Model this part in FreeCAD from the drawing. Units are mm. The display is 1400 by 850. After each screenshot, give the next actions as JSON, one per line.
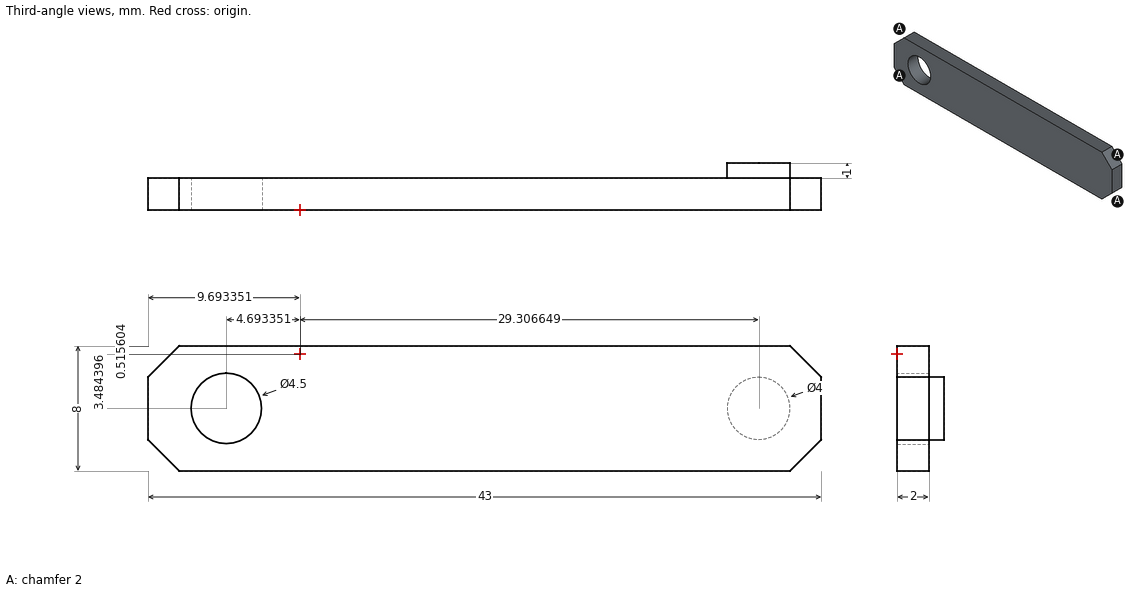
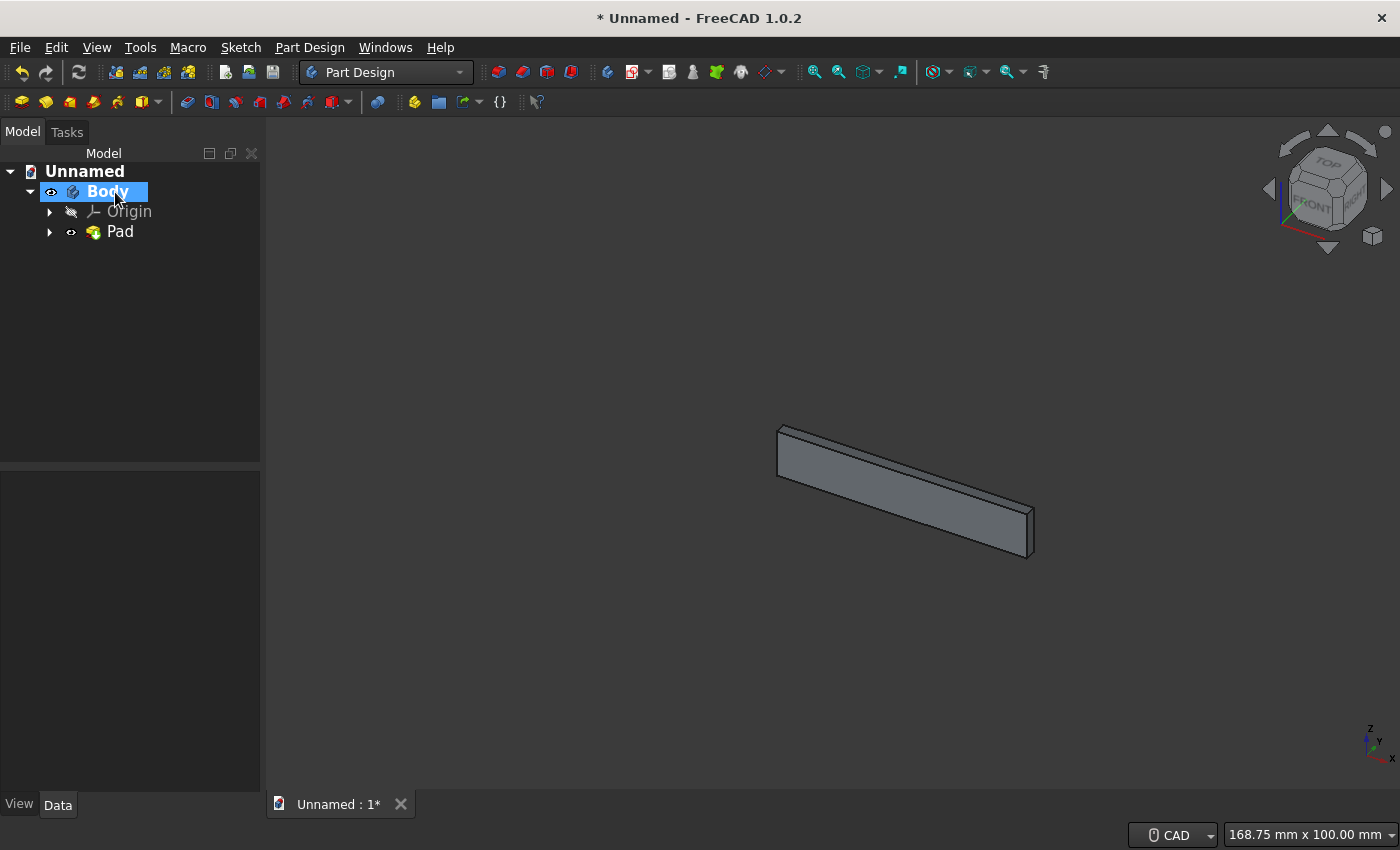
{"action": "left_click", "coordinate": [816, 72]}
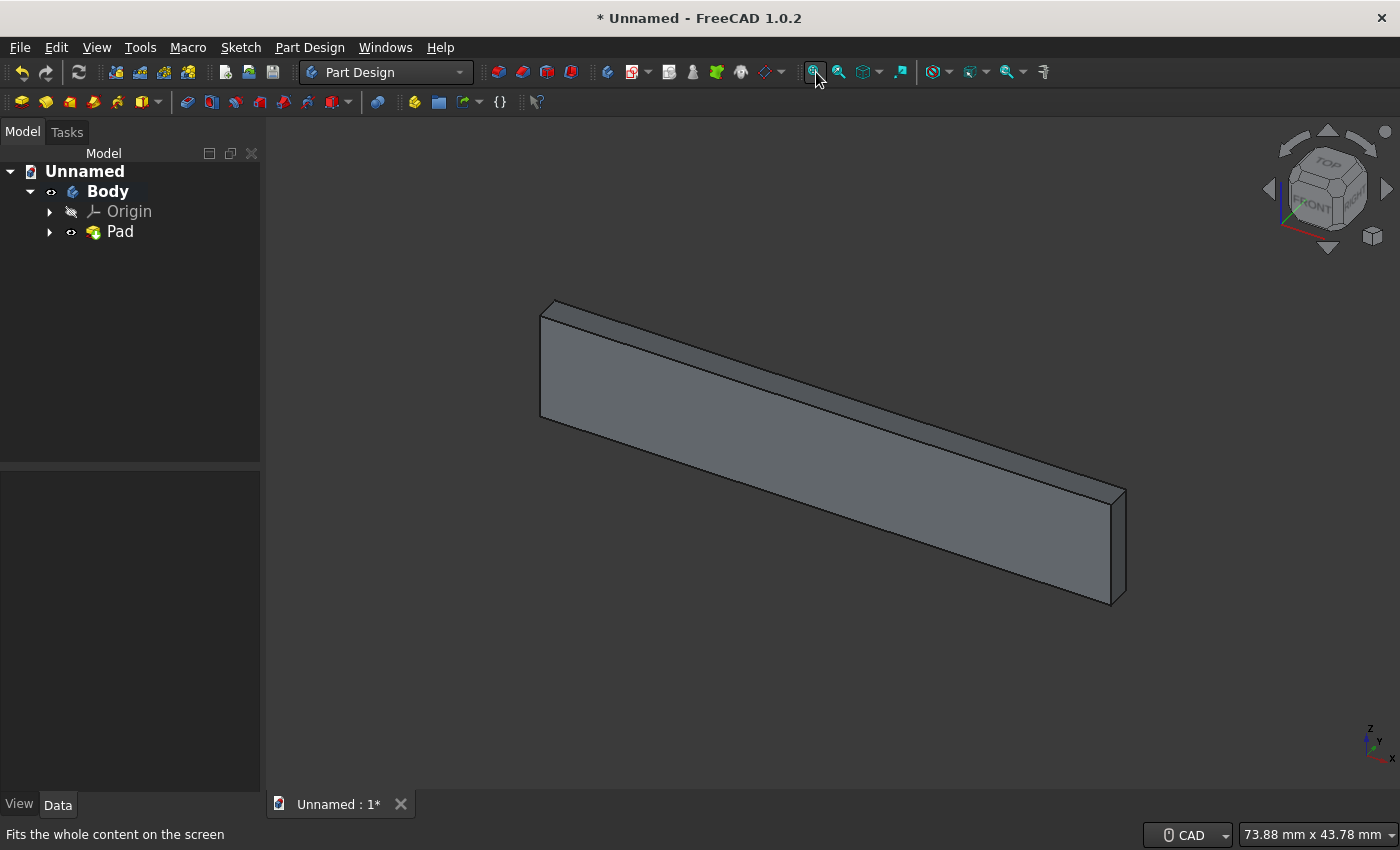
{"action": "key", "text": "4"}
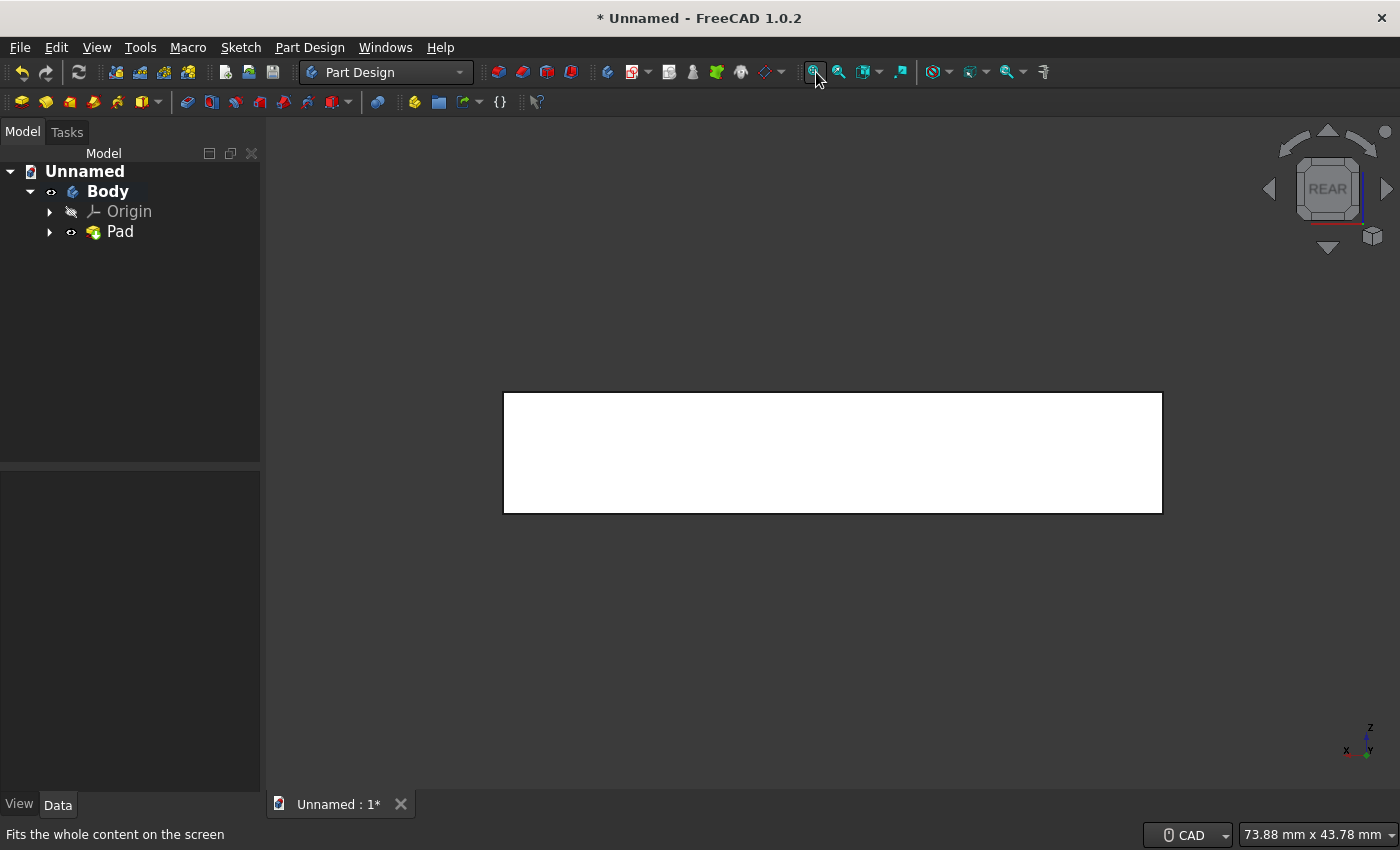
{"action": "left_click", "coordinate": [644, 452]}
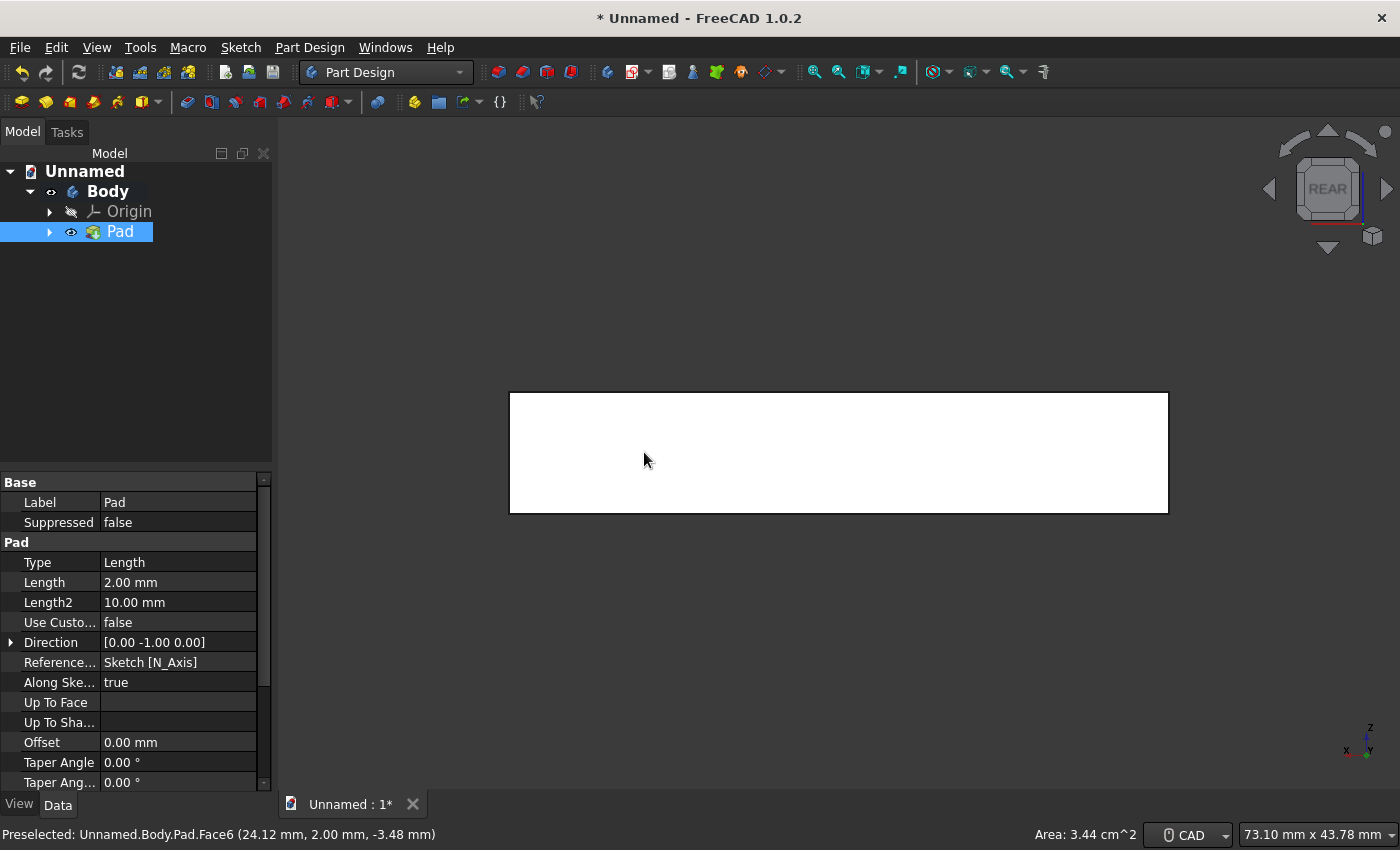
{"action": "left_click", "coordinate": [632, 72]}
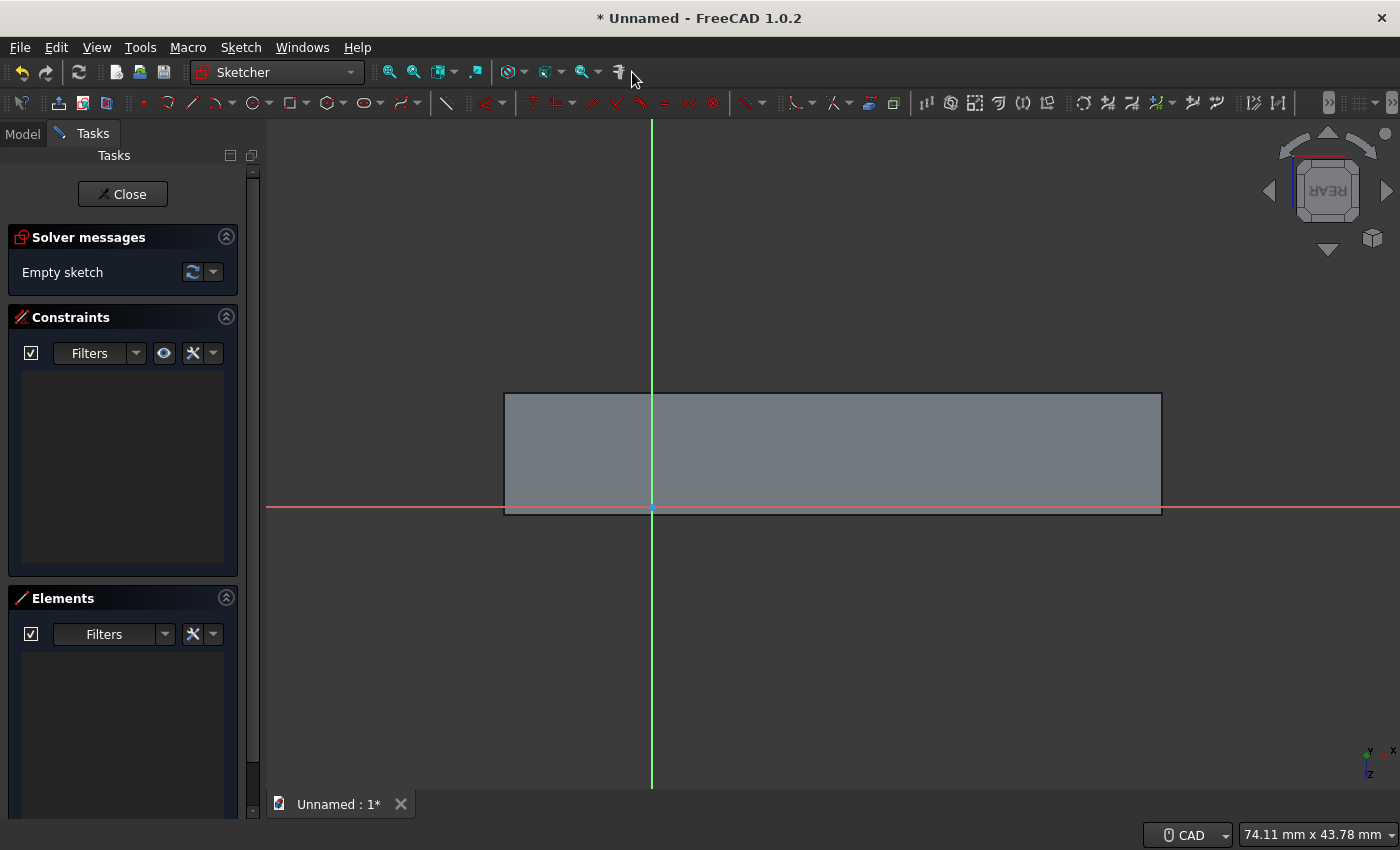
{"action": "scroll", "coordinate": [557, 466], "scroll_direction": "up", "scroll_amount": 8}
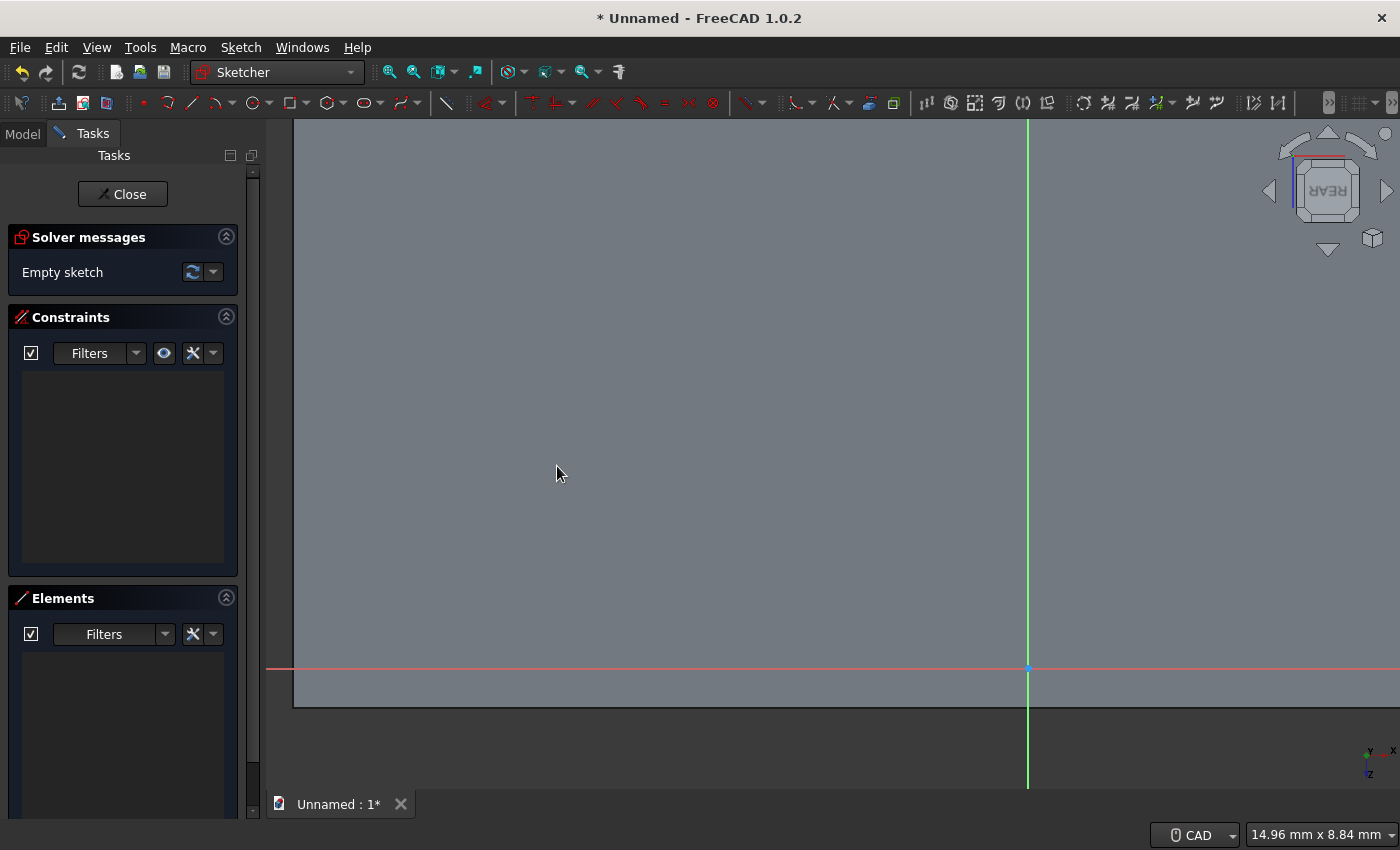
{"action": "left_click", "coordinate": [254, 104]}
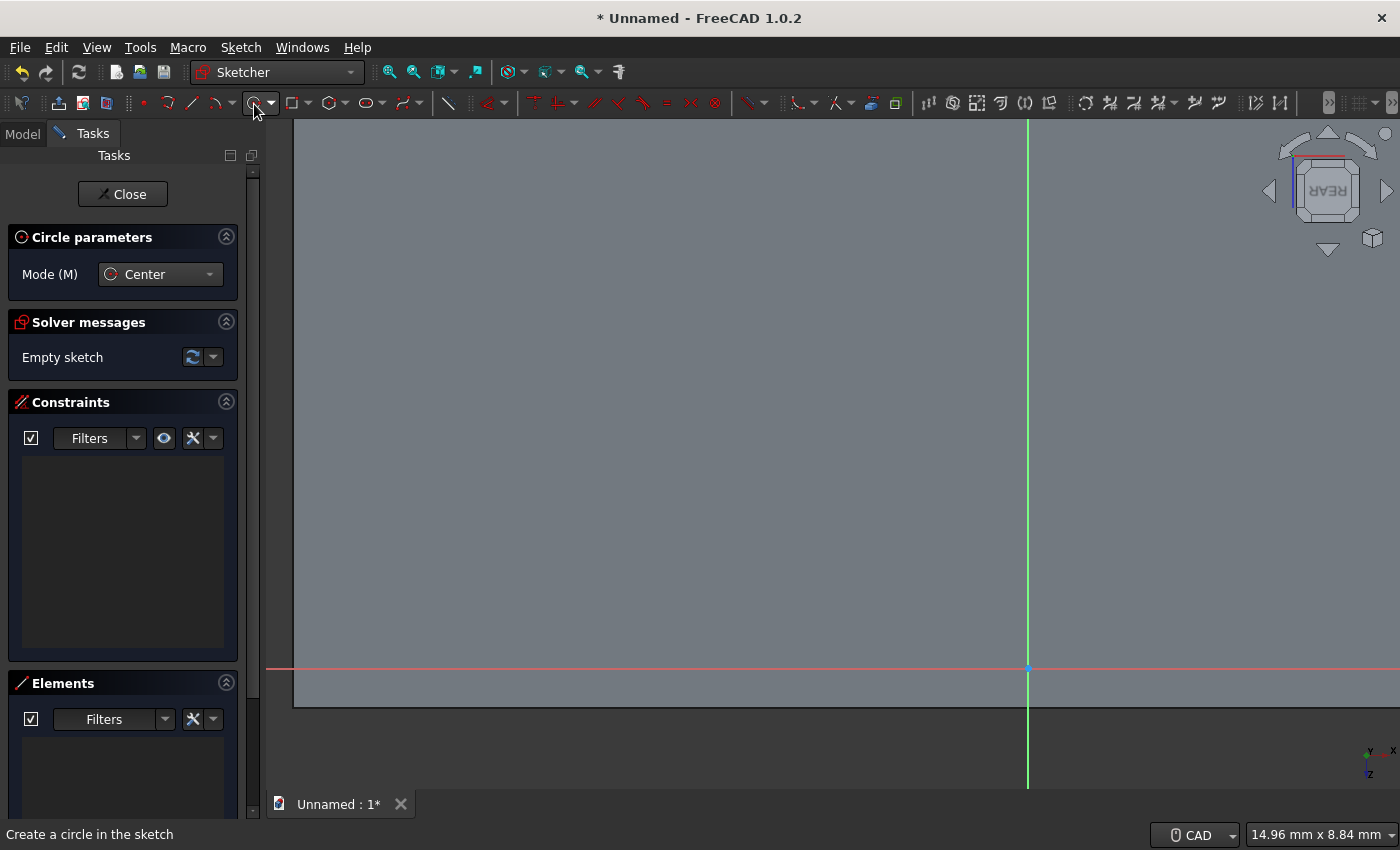
{"action": "left_click", "coordinate": [672, 405]}
{"action": "left_click", "coordinate": [793, 284]}
{"action": "key", "text": "Escape"}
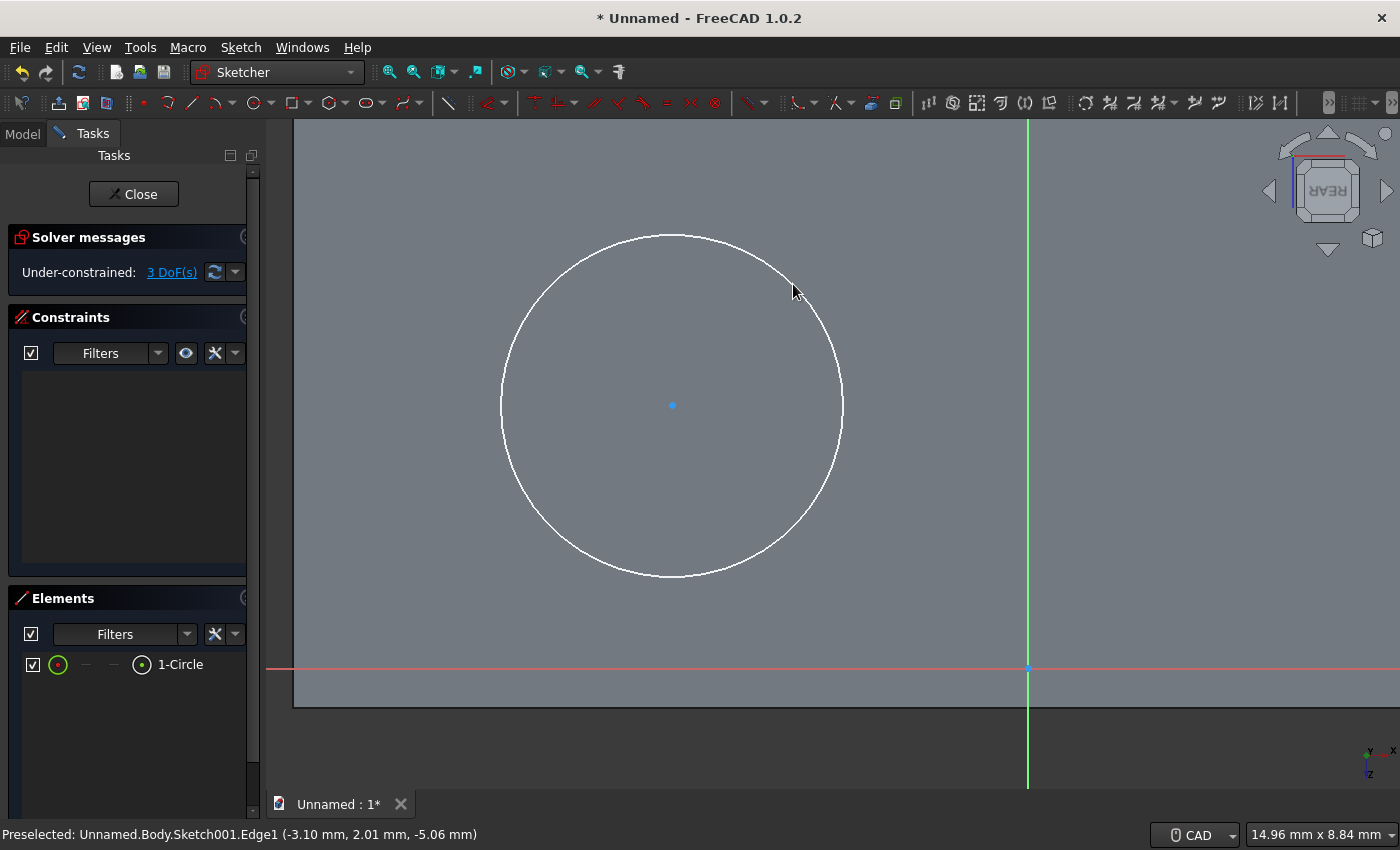
{"action": "left_click", "coordinate": [488, 104]}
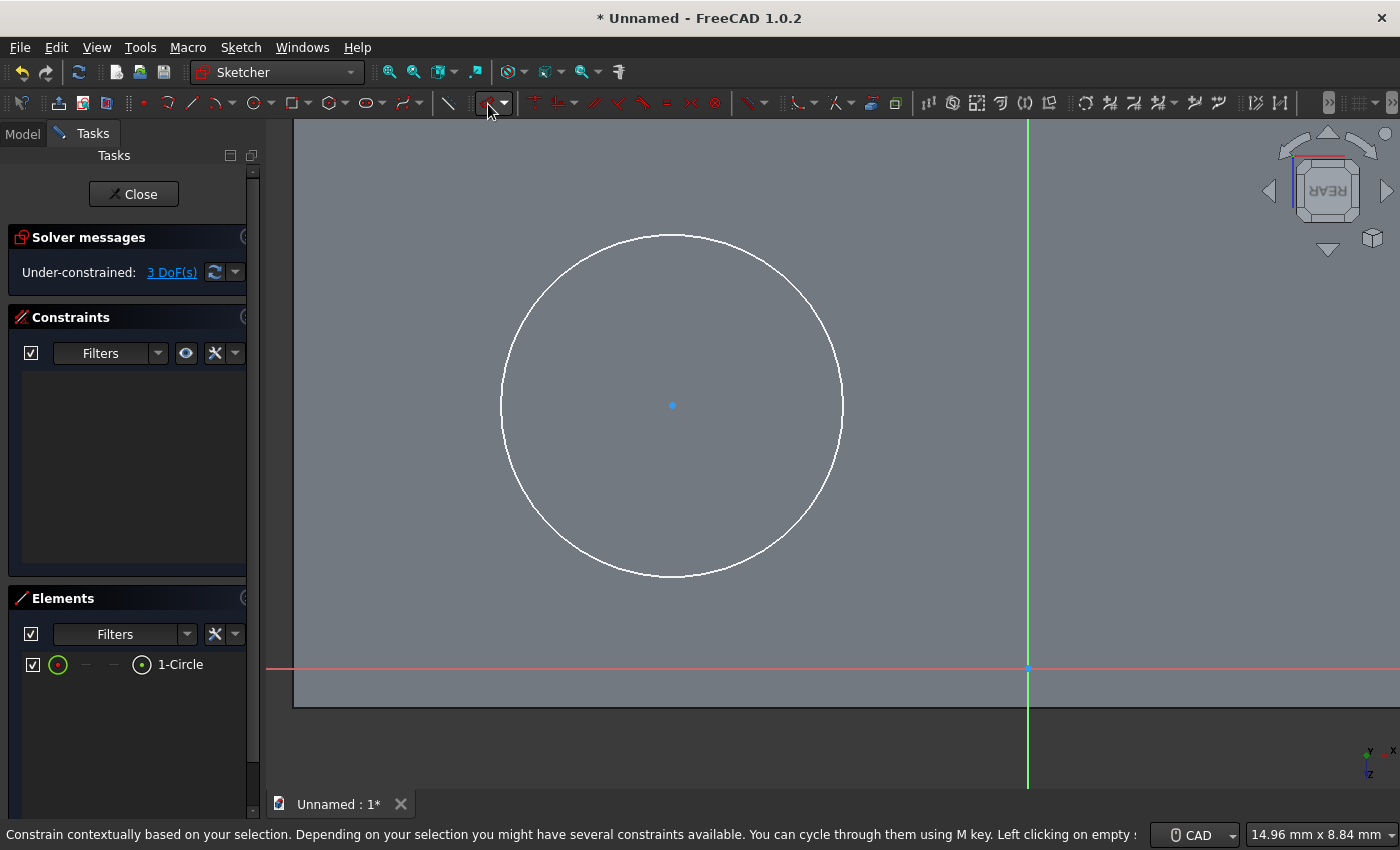
{"action": "left_click", "coordinate": [793, 285]}
{"action": "left_click", "coordinate": [816, 262]}